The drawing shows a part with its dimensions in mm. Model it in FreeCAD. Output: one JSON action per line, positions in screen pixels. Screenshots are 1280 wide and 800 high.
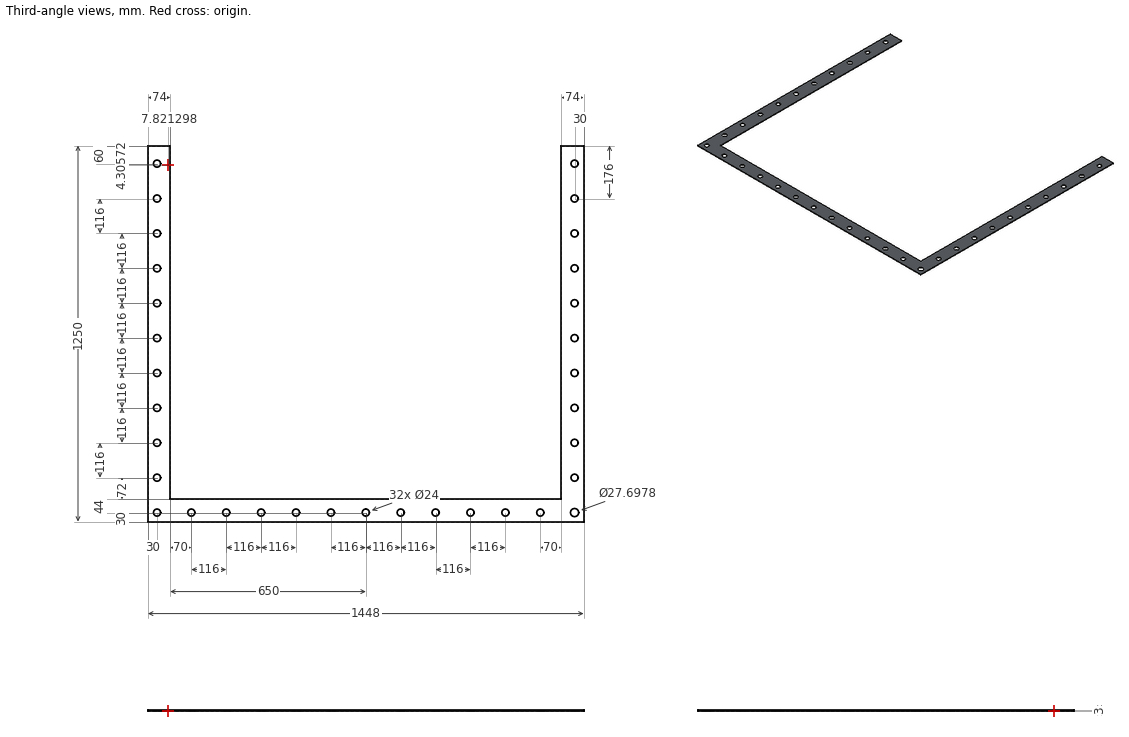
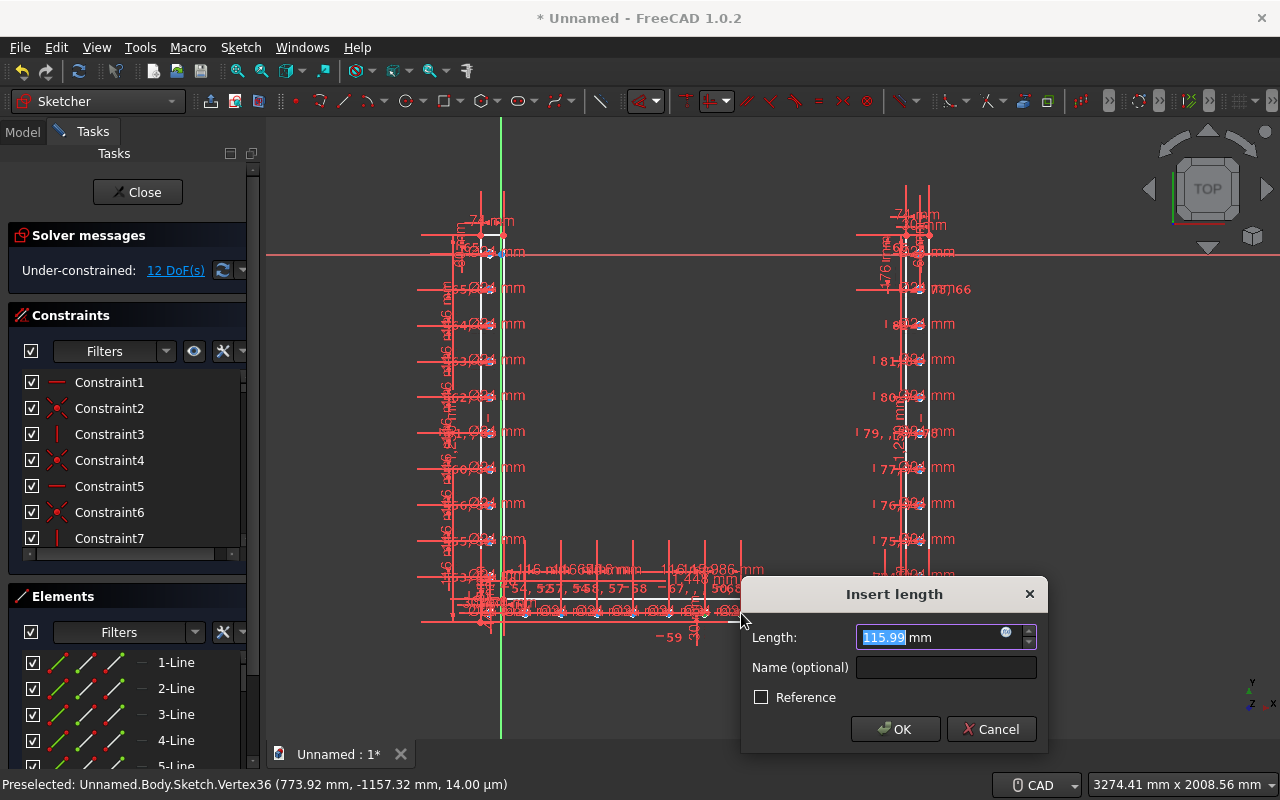
{"action": "type", "text": "116"}
{"action": "key", "text": "Return"}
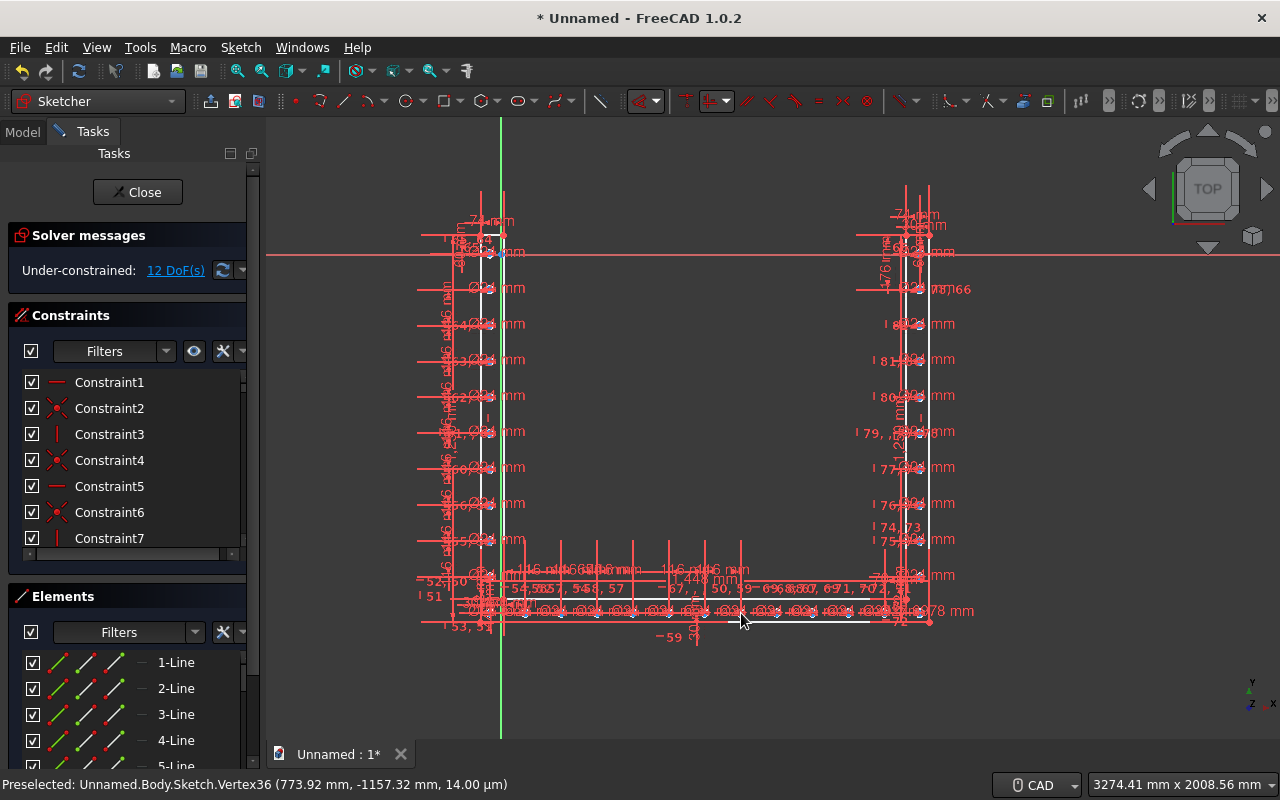
{"action": "left_click", "coordinate": [741, 613]}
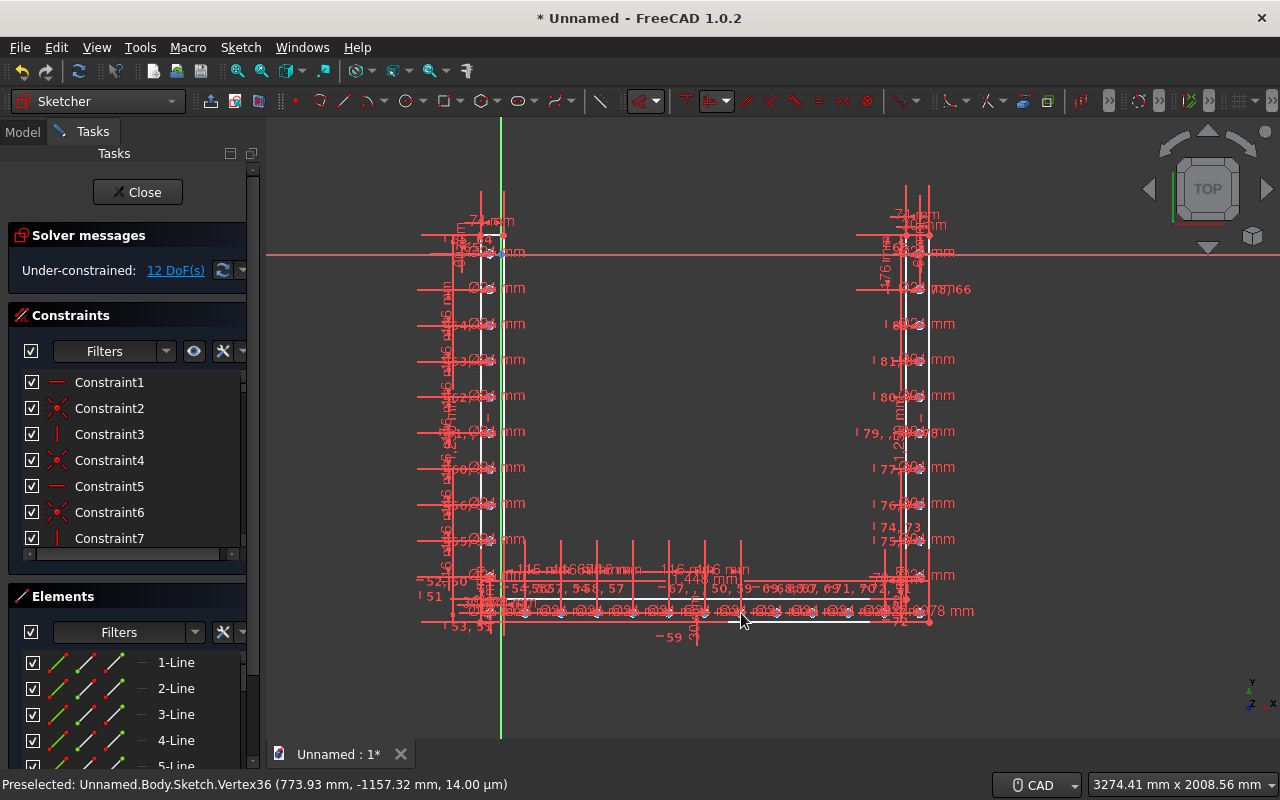
{"action": "left_click", "coordinate": [777, 613]}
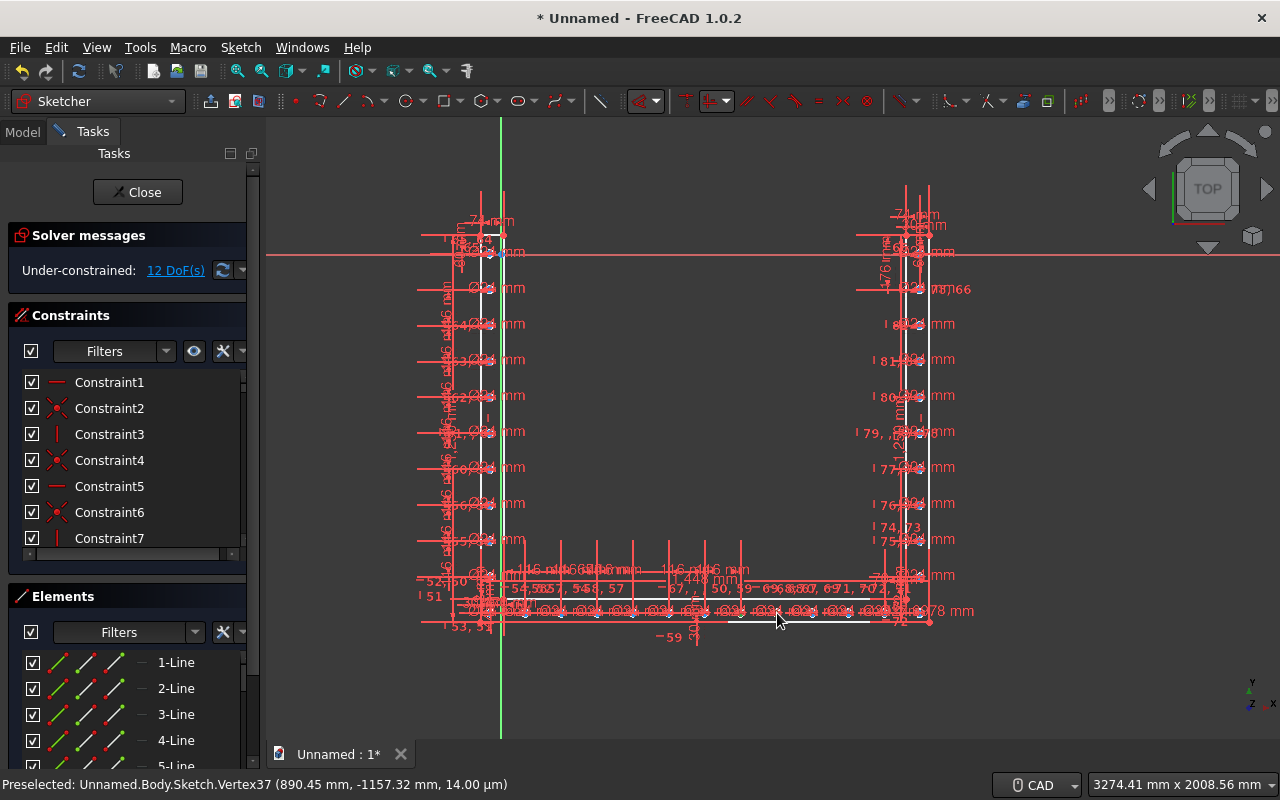
{"action": "left_click", "coordinate": [658, 102]}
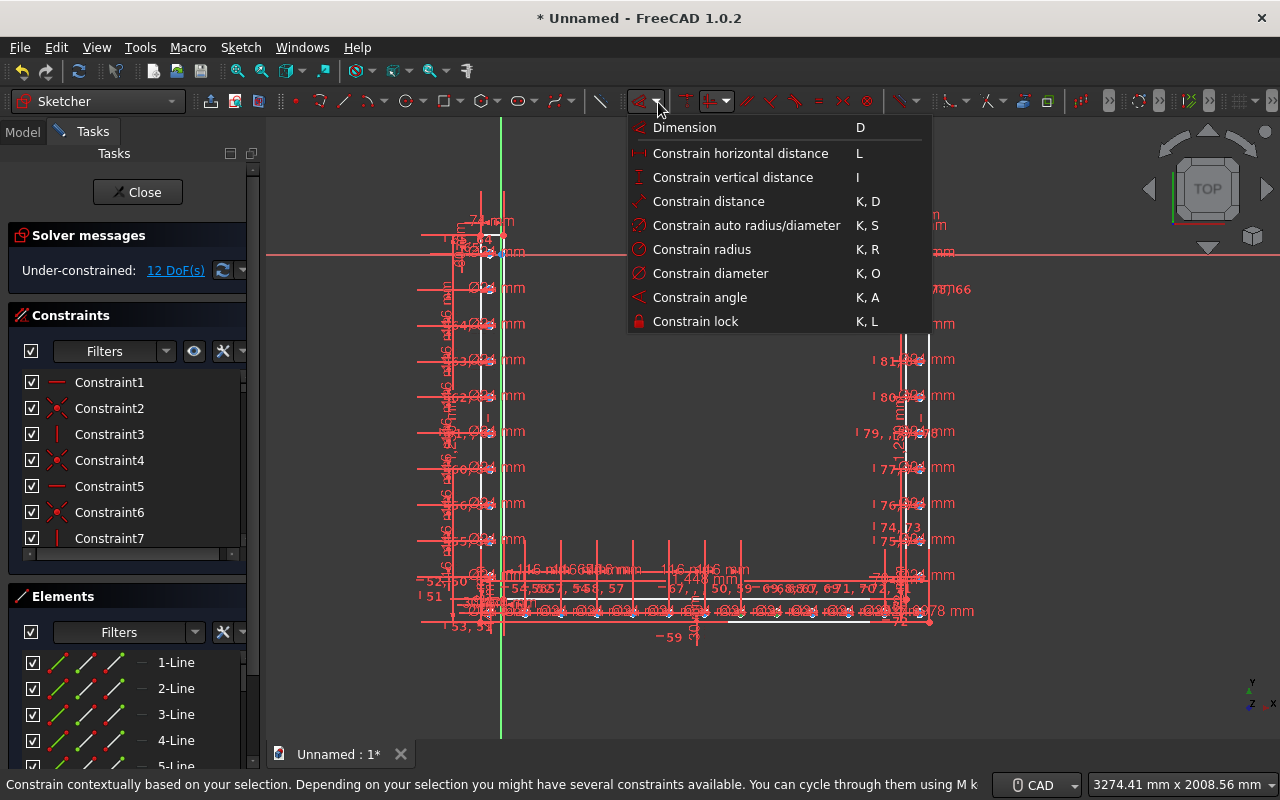
{"action": "left_click", "coordinate": [780, 153]}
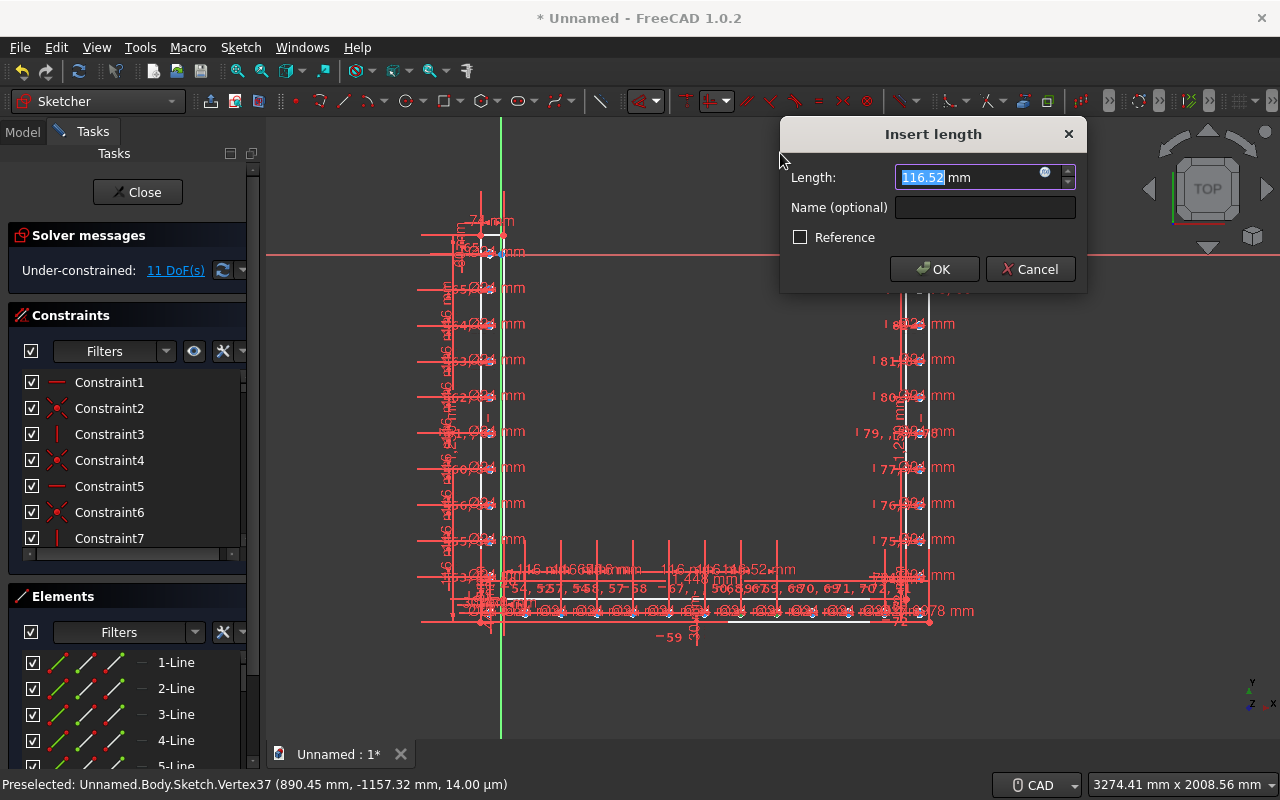
{"action": "type", "text": "116"}
{"action": "key", "text": "Return"}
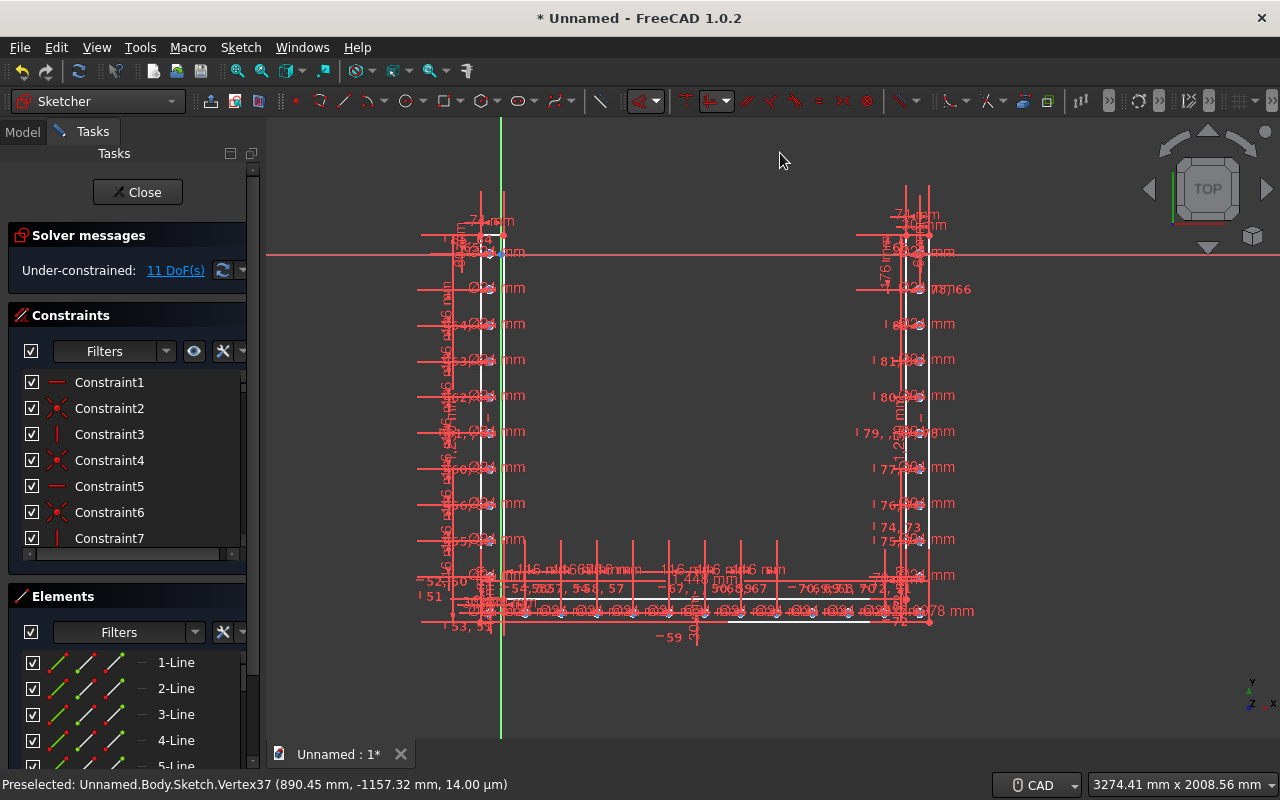
{"action": "left_click", "coordinate": [777, 613]}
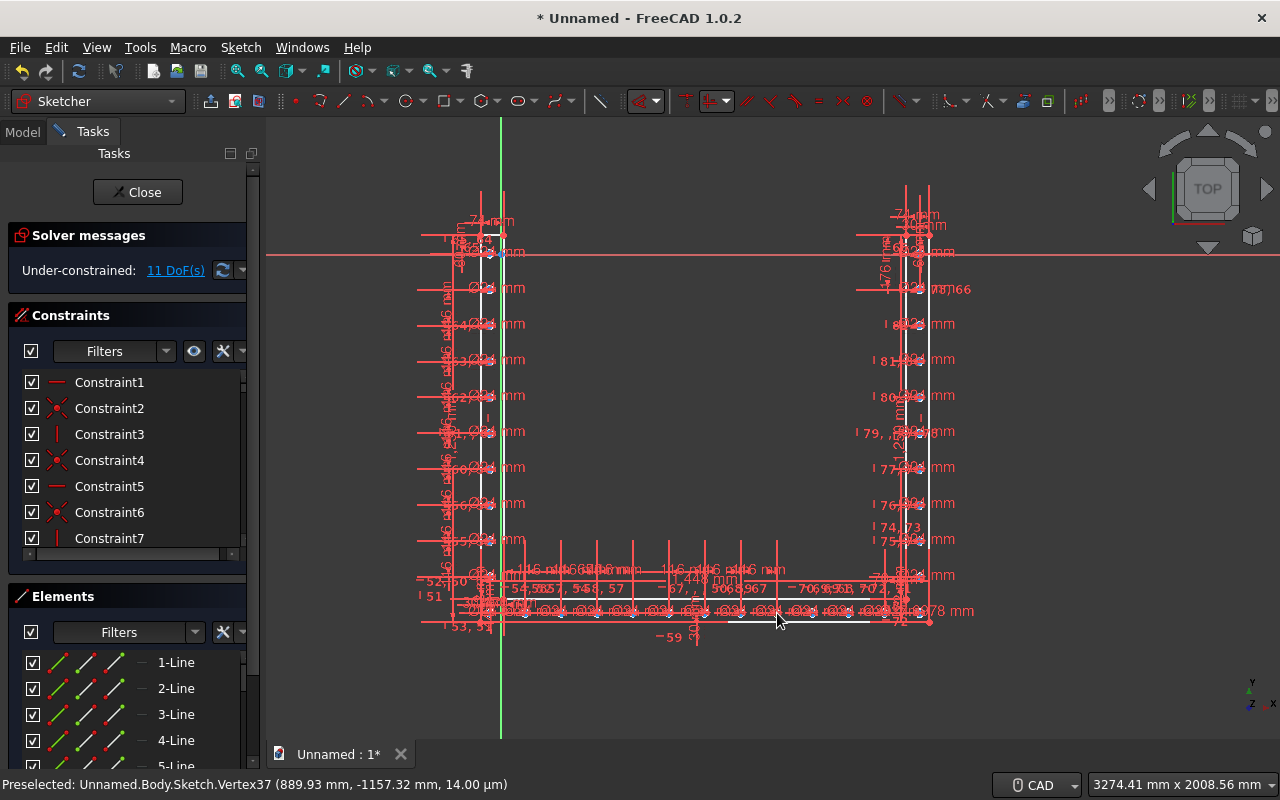
{"action": "left_click", "coordinate": [812, 613]}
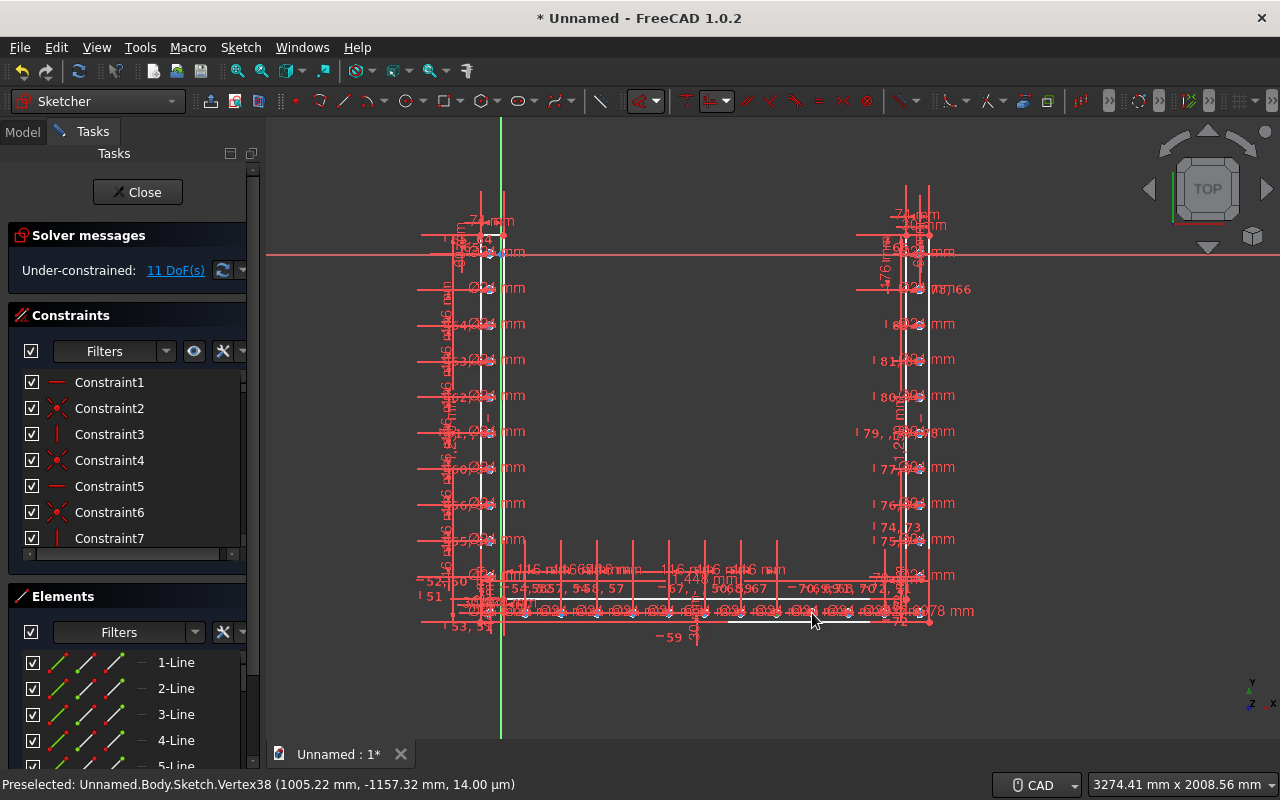
{"action": "left_click", "coordinate": [658, 102]}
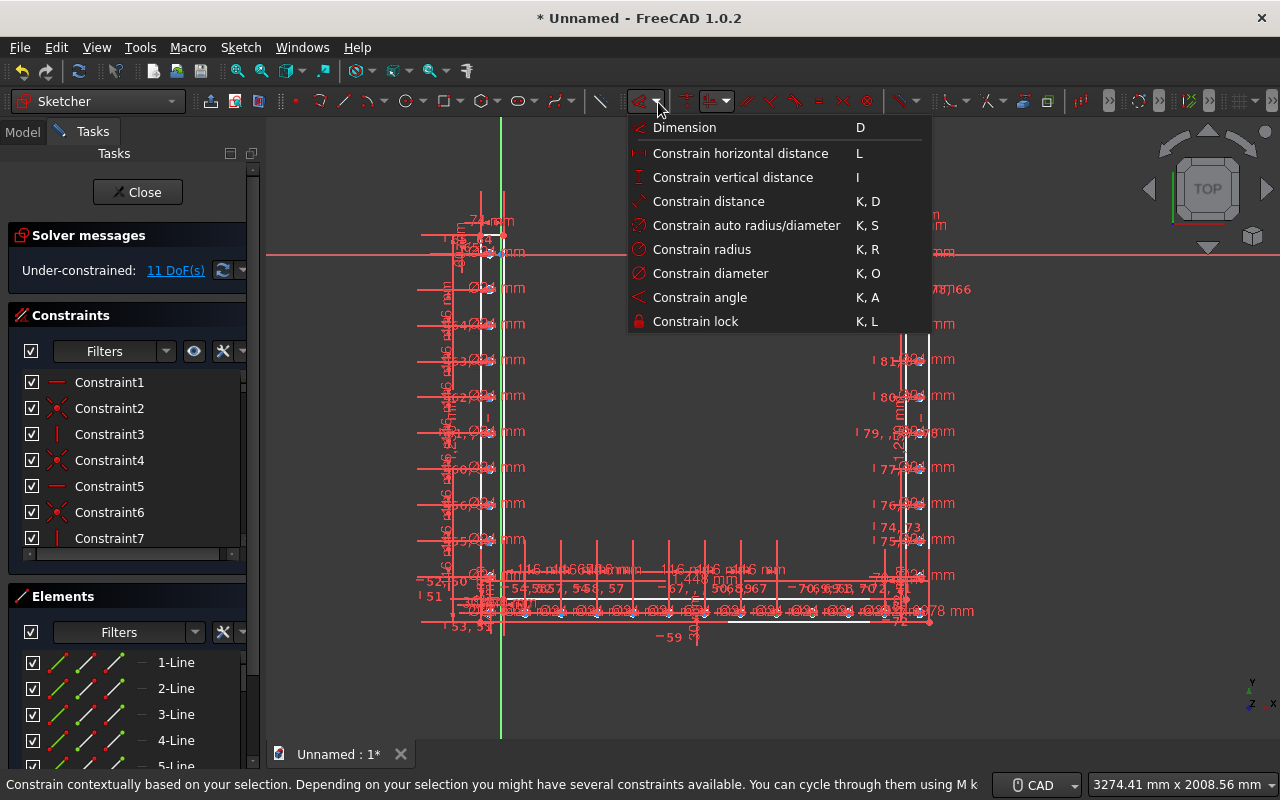
{"action": "left_click", "coordinate": [780, 153]}